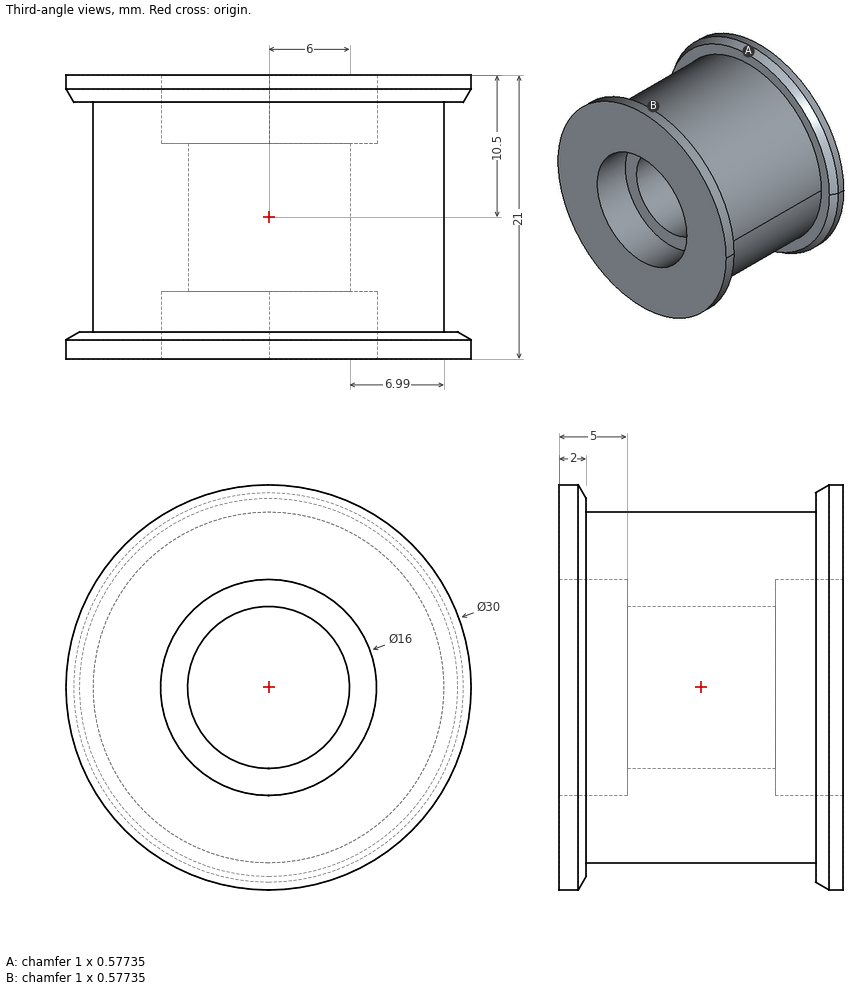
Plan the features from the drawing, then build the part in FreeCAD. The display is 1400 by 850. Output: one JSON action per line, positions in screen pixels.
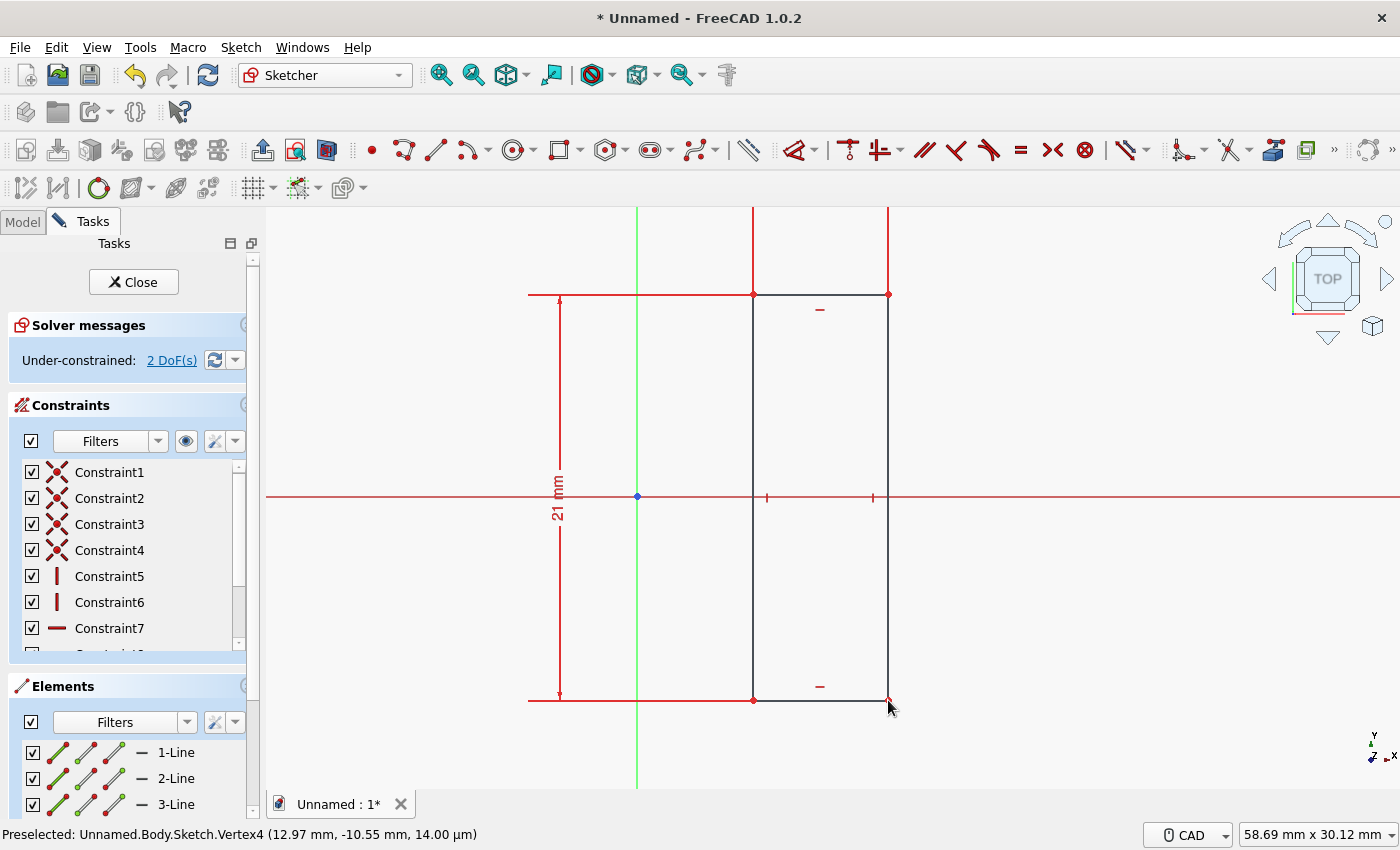
{"action": "left_click", "coordinate": [794, 150]}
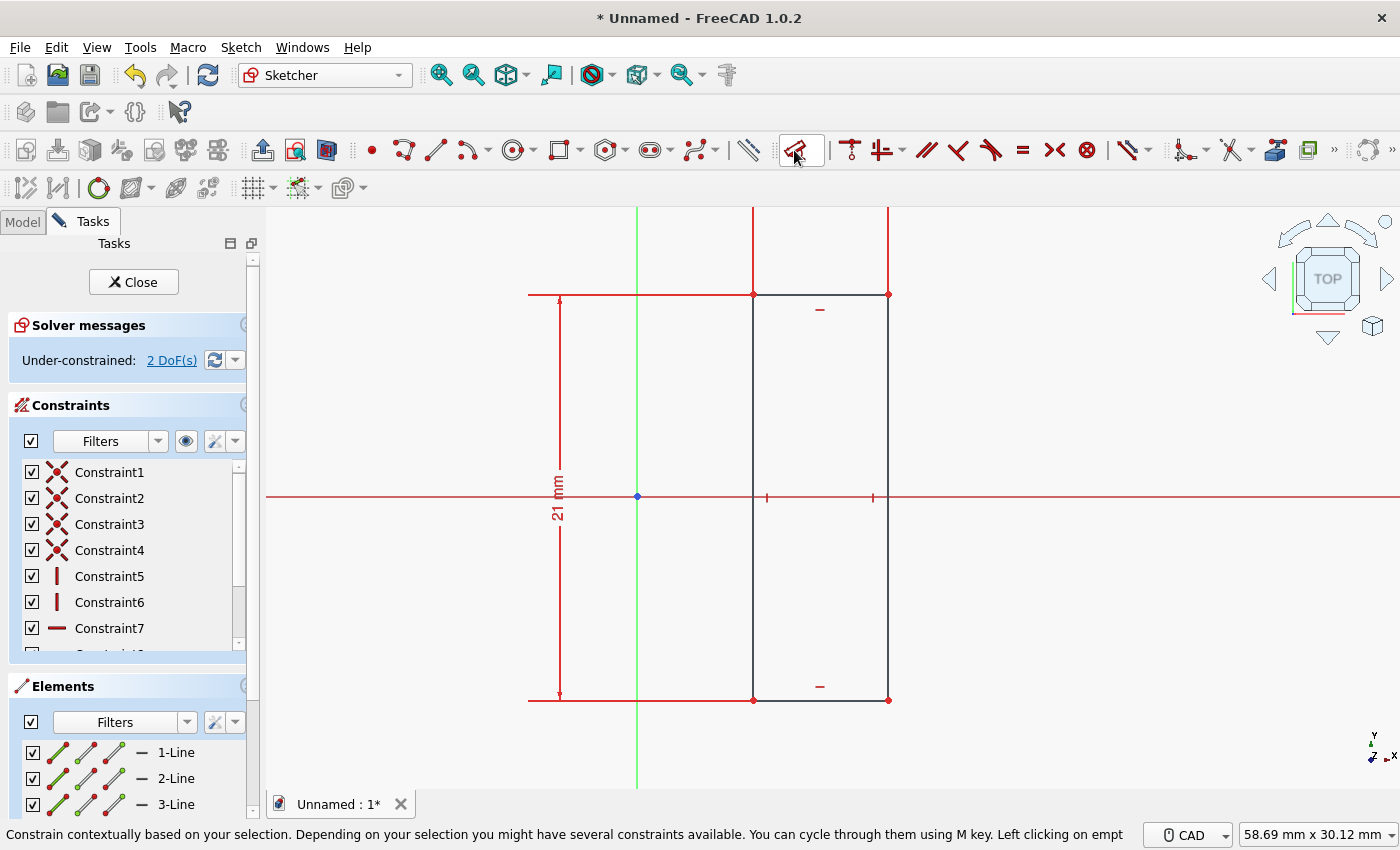
{"action": "left_click", "coordinate": [753, 295]}
{"action": "left_click", "coordinate": [695, 261]}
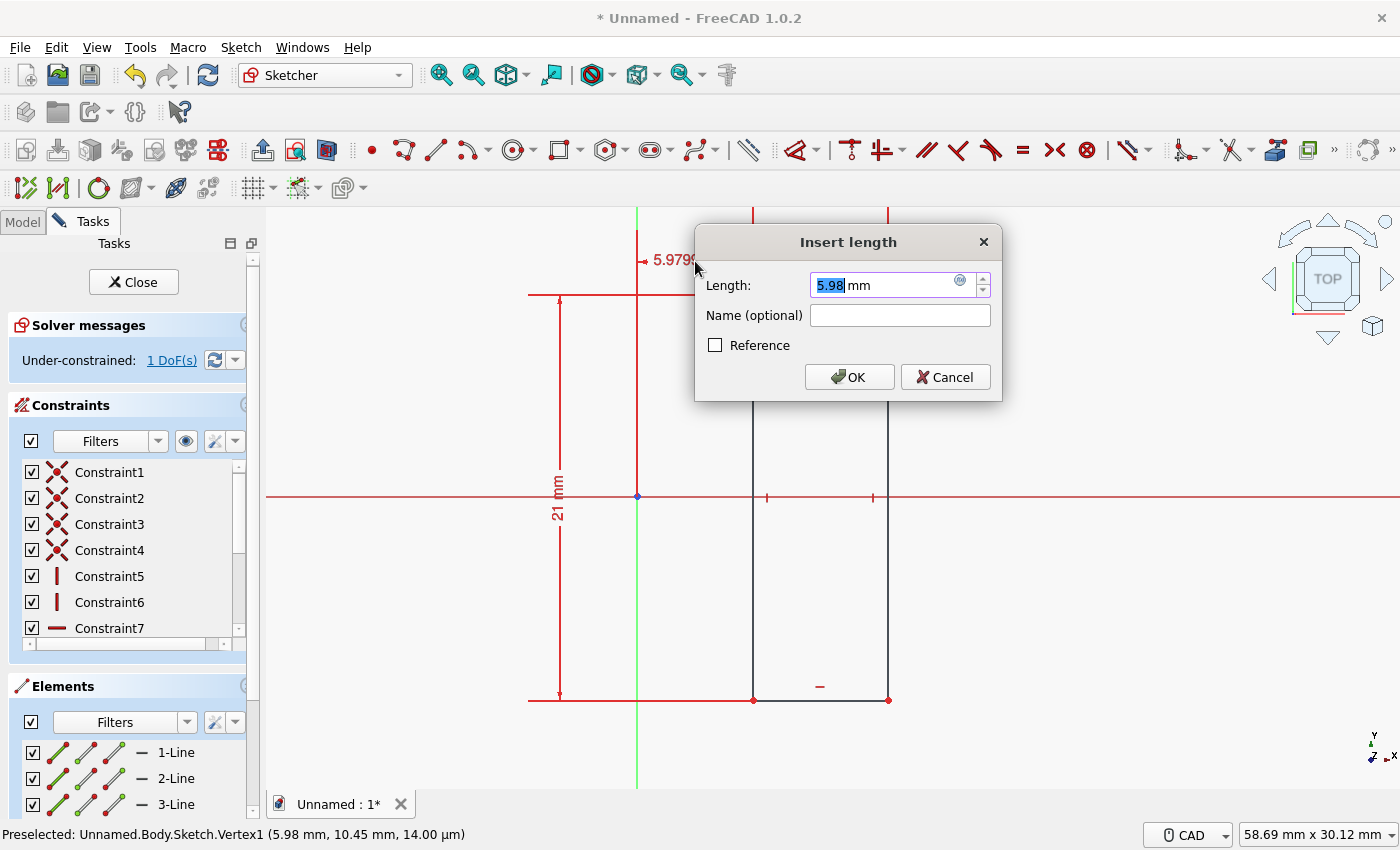
{"action": "type", "text": "6"}
{"action": "key", "text": "Return"}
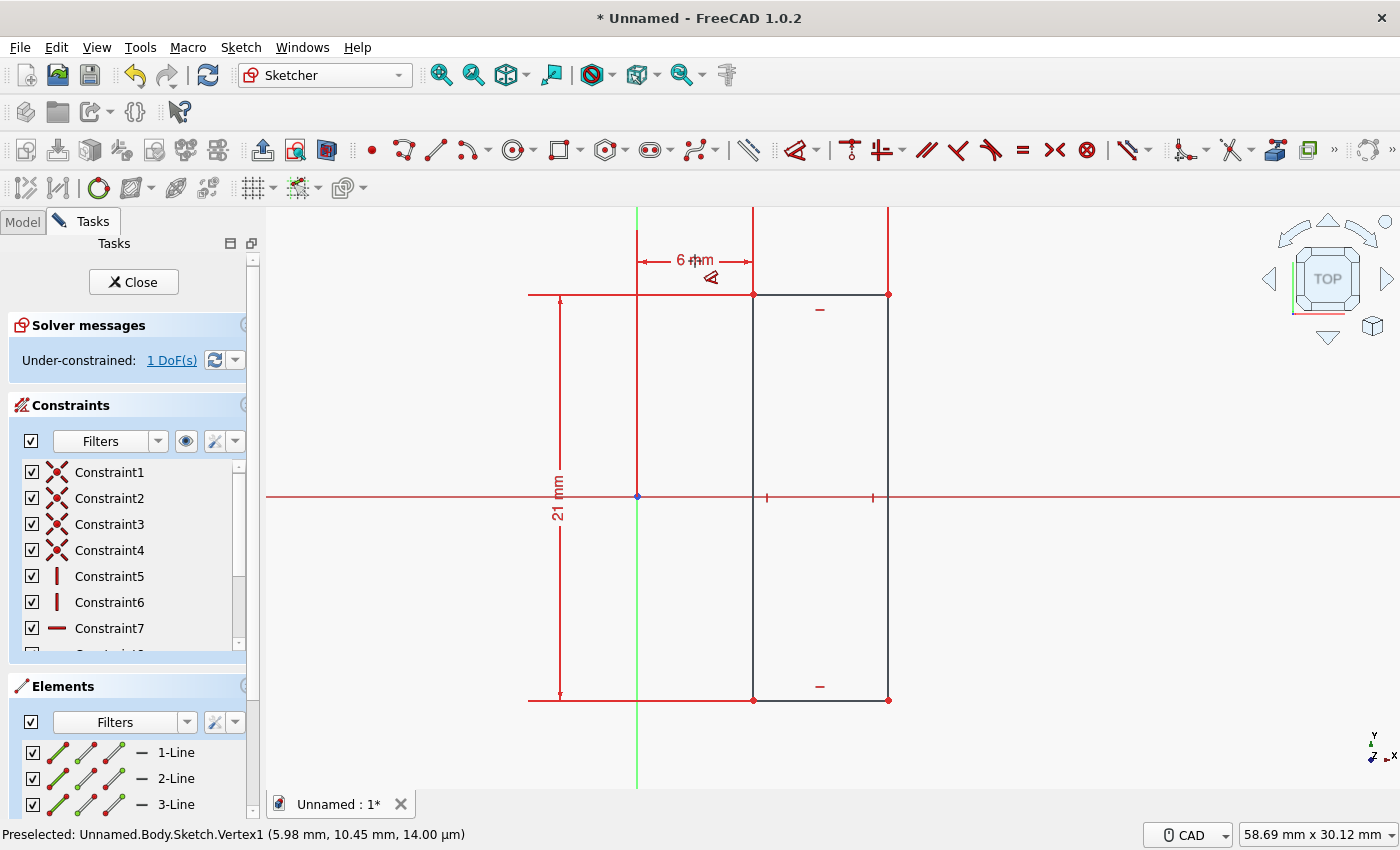
{"action": "left_click", "coordinate": [753, 295]}
{"action": "left_click", "coordinate": [603, 396]}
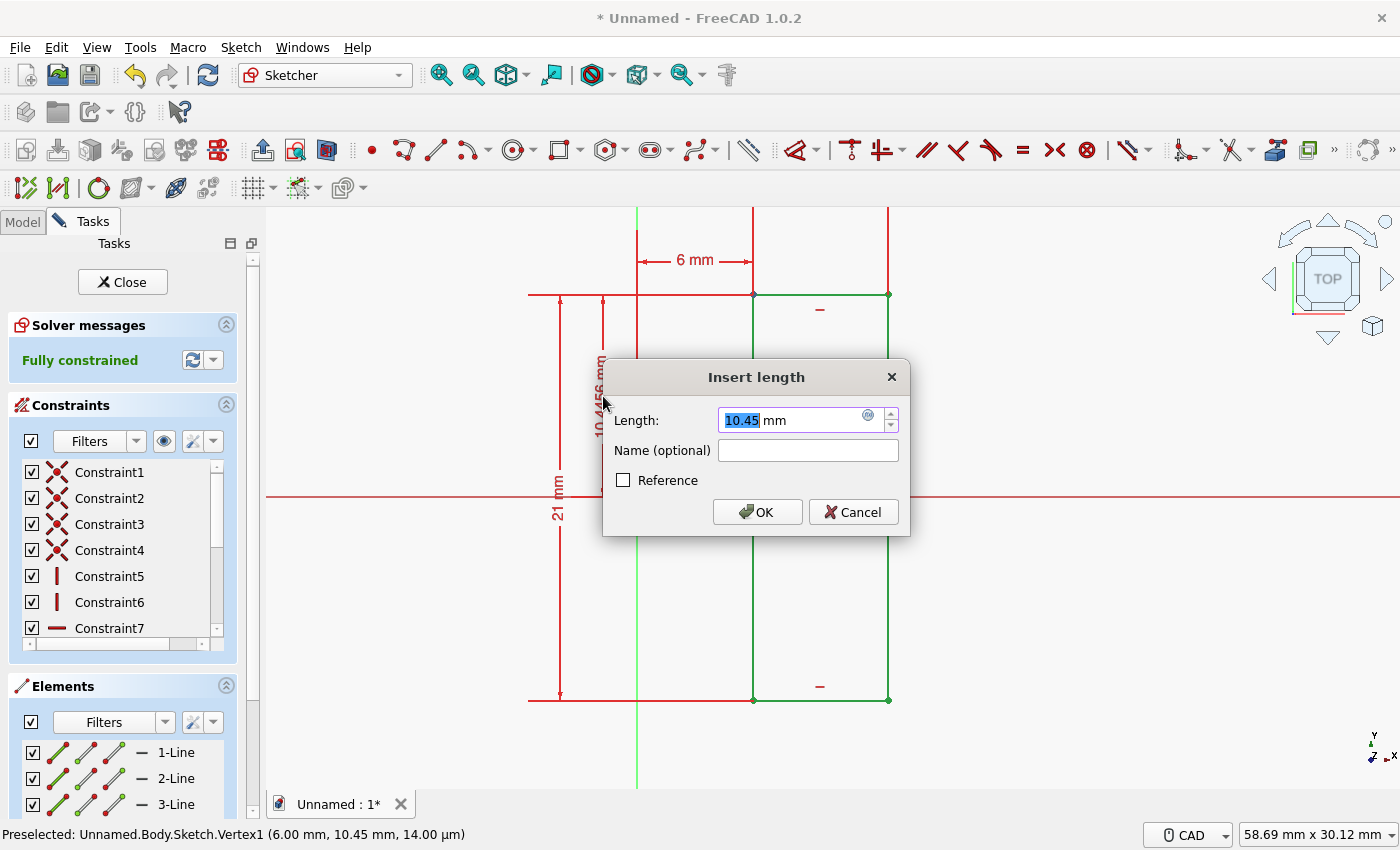
{"action": "type", "text": "10.5"}
{"action": "key", "text": "Return"}
{"action": "key", "text": "Escape"}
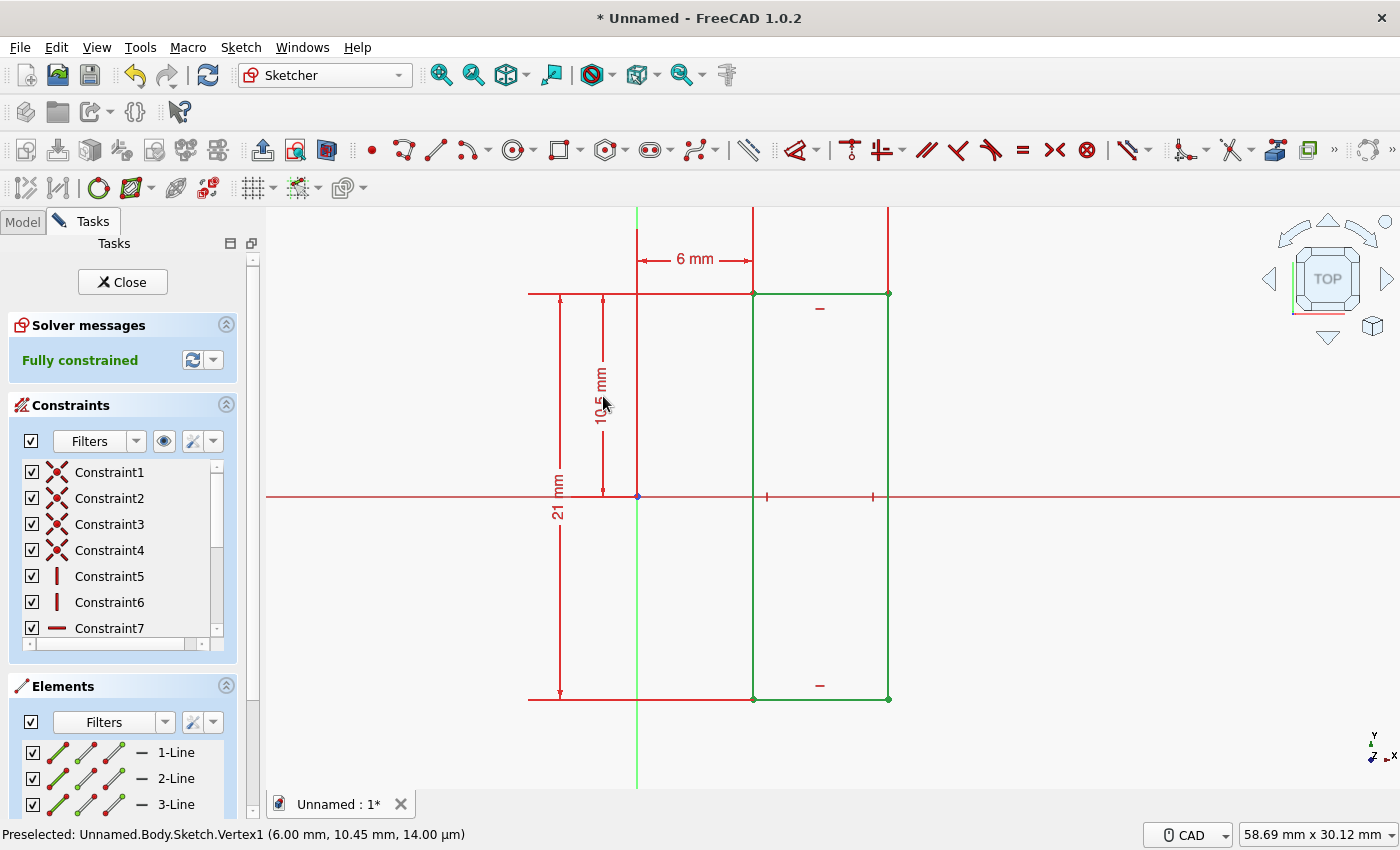
{"action": "left_click", "coordinate": [123, 282]}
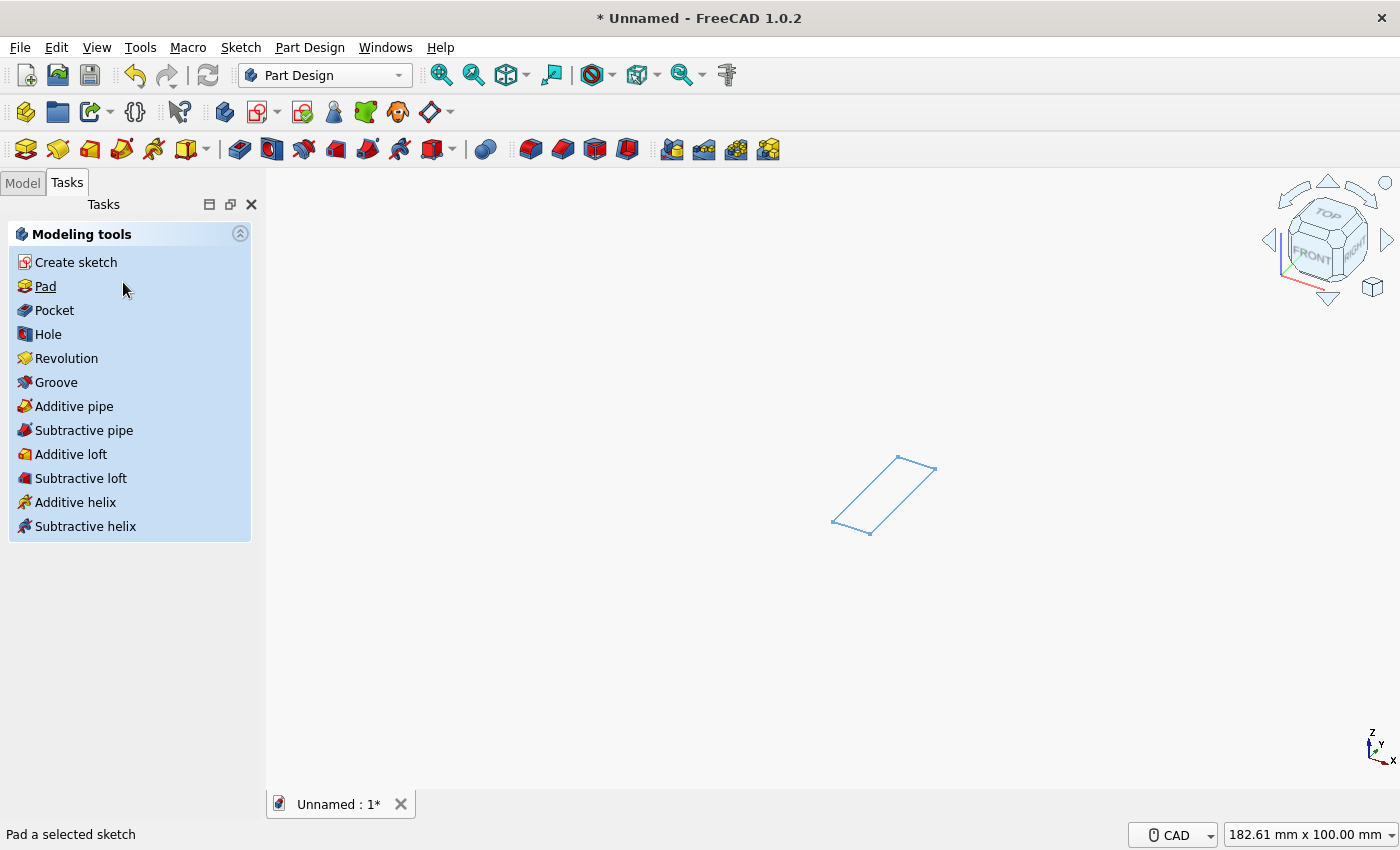
{"action": "left_click", "coordinate": [58, 150]}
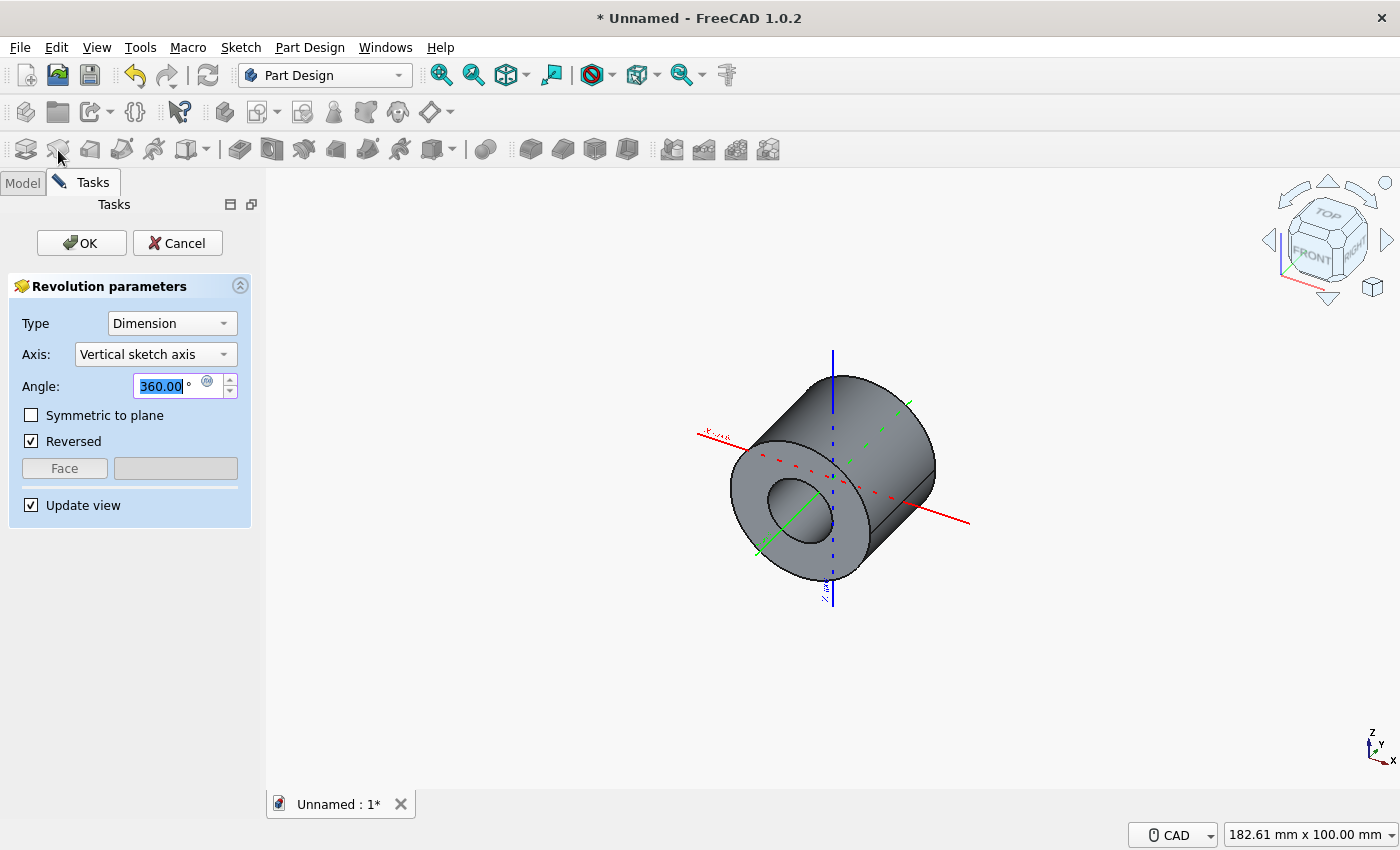
{"action": "left_click", "coordinate": [82, 243]}